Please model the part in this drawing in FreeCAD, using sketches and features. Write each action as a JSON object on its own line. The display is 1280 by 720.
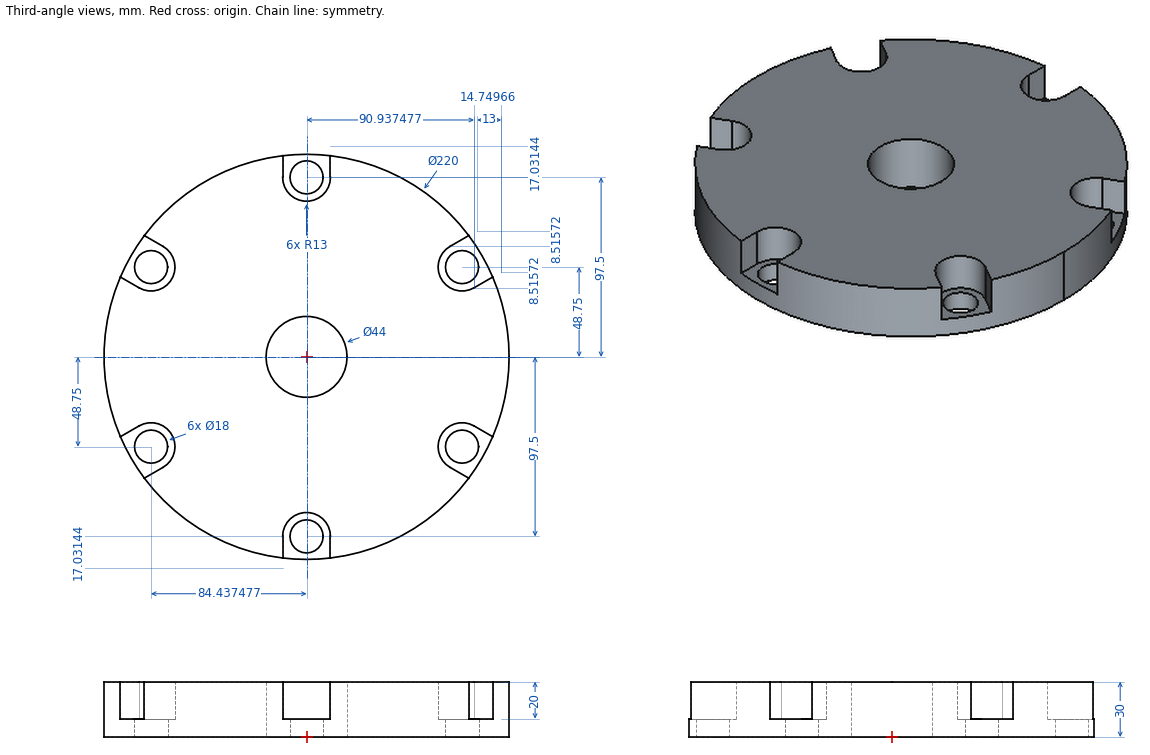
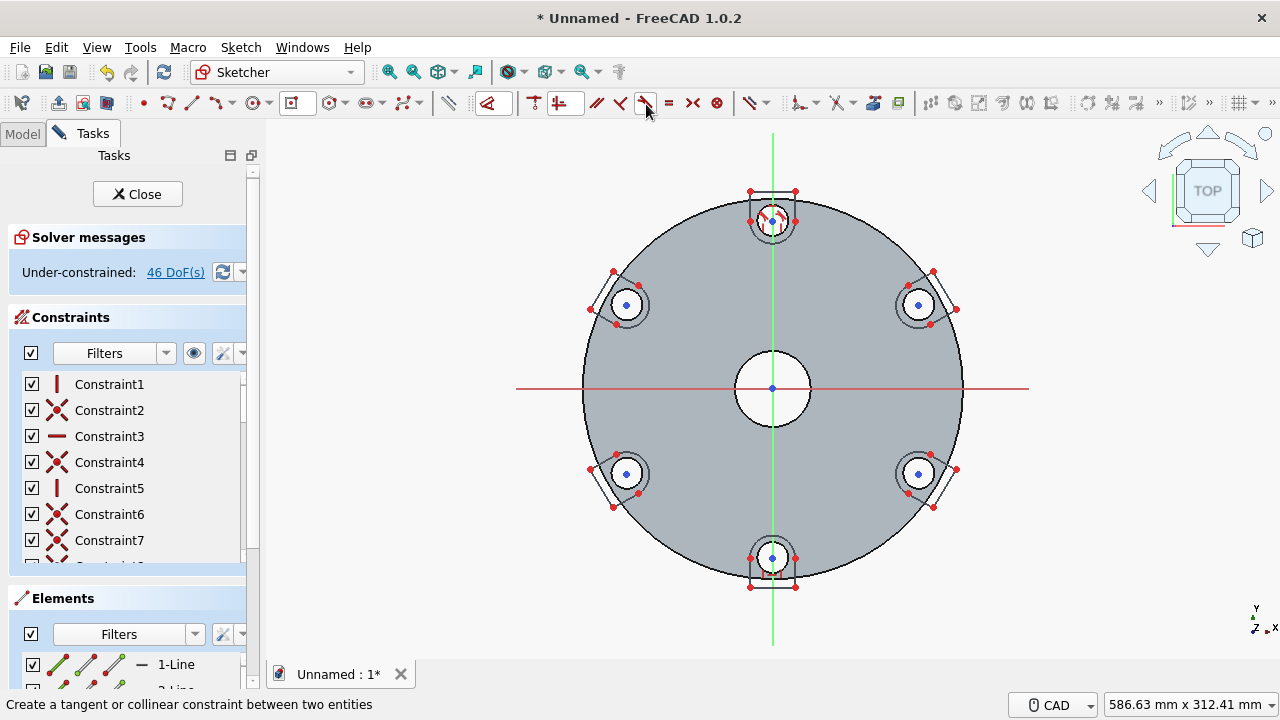
{"action": "scroll", "coordinate": [938, 320], "scroll_direction": "up", "scroll_amount": 3}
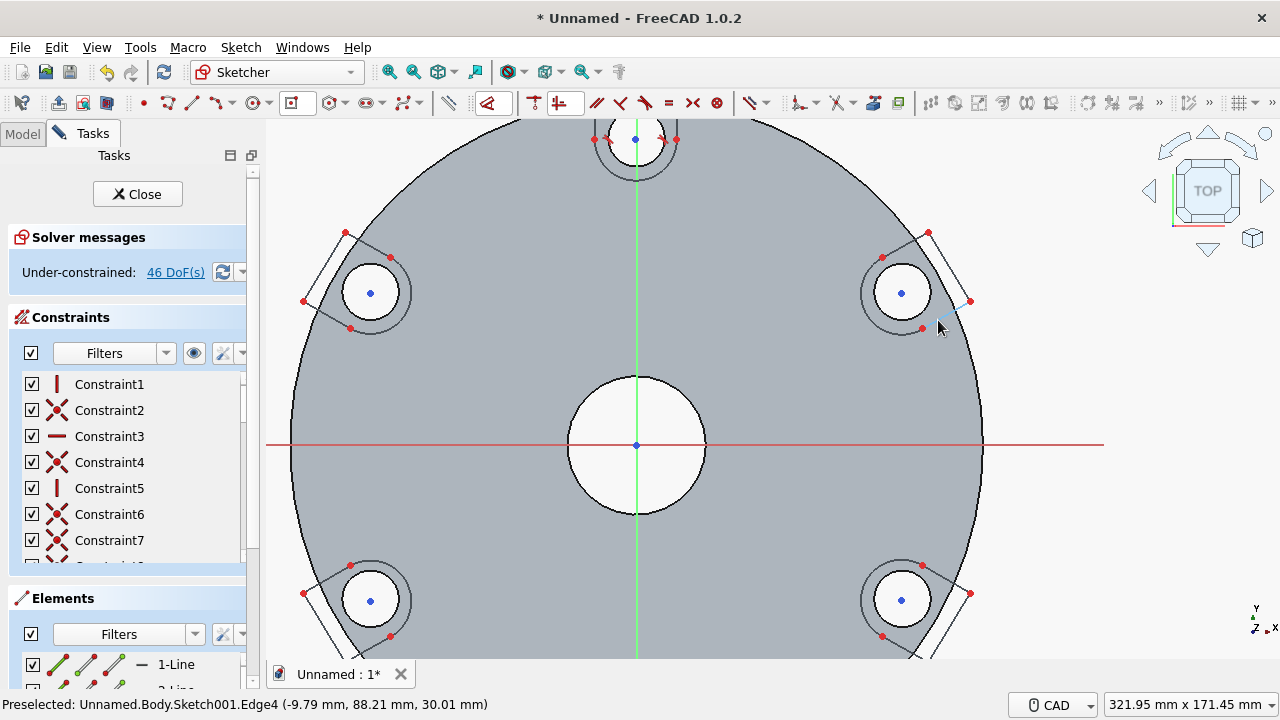
{"action": "left_click", "coordinate": [937, 321]}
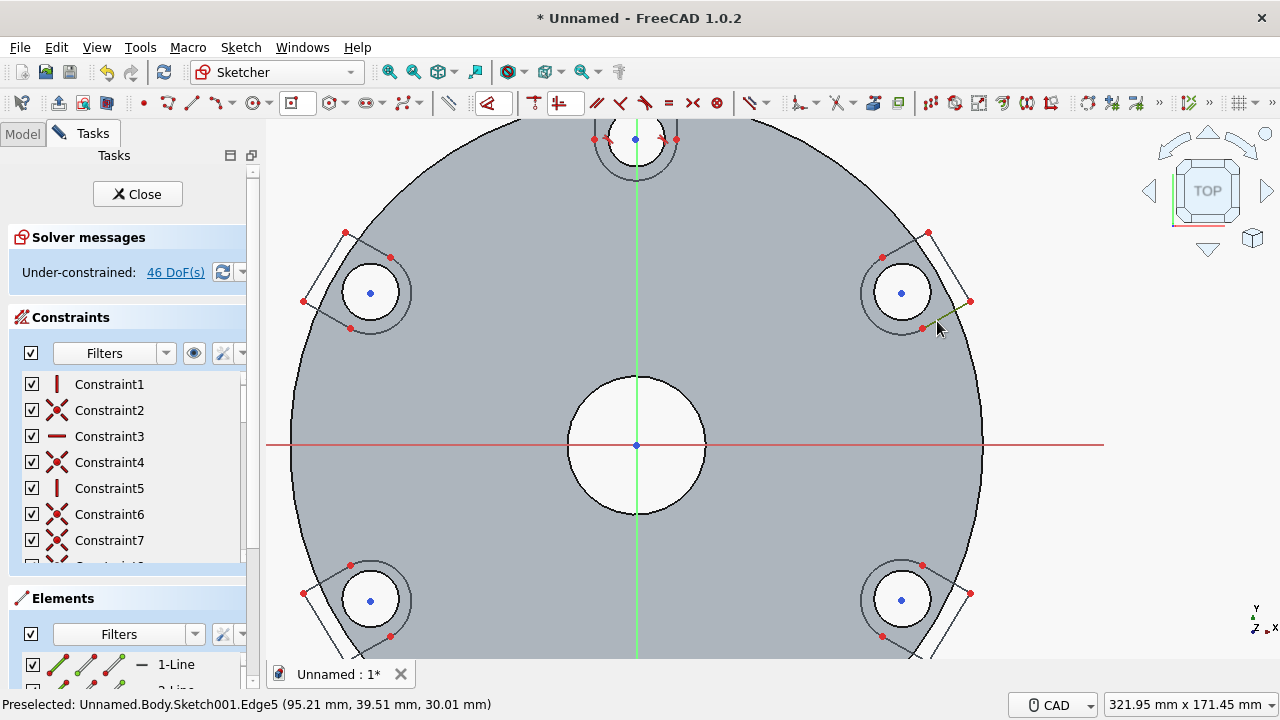
{"action": "left_click", "coordinate": [861, 289]}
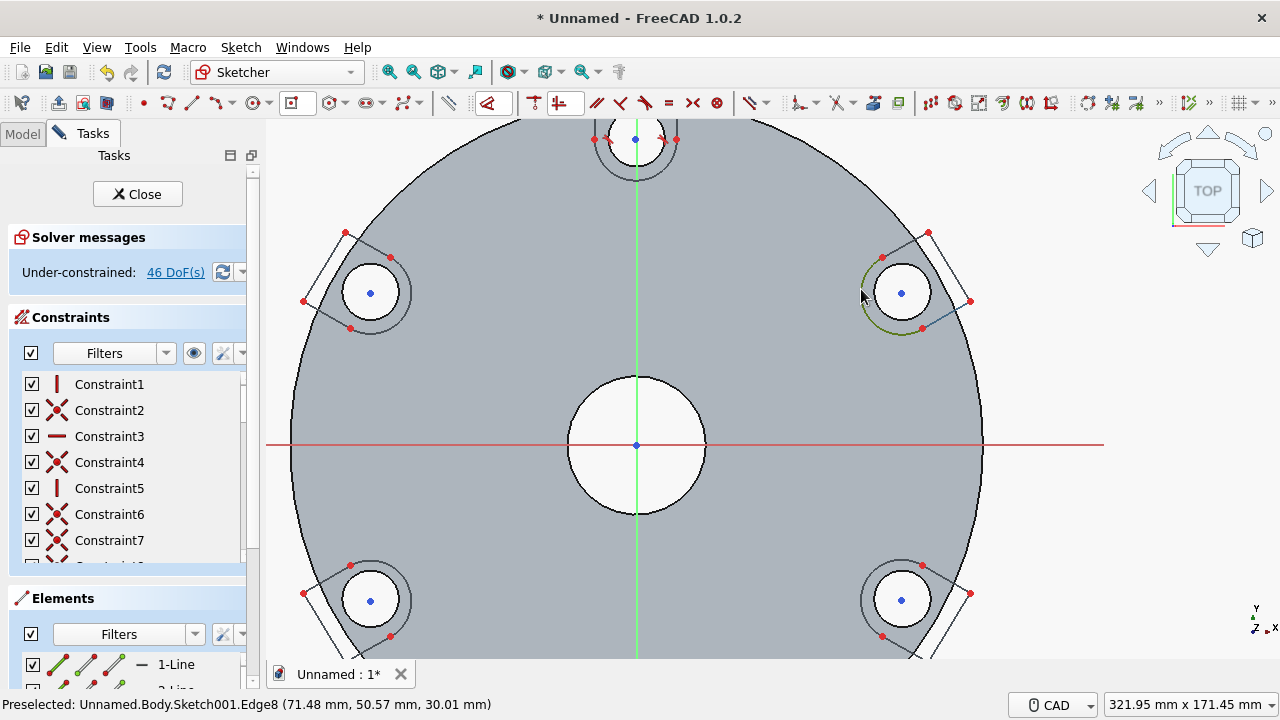
{"action": "key", "text": "t"}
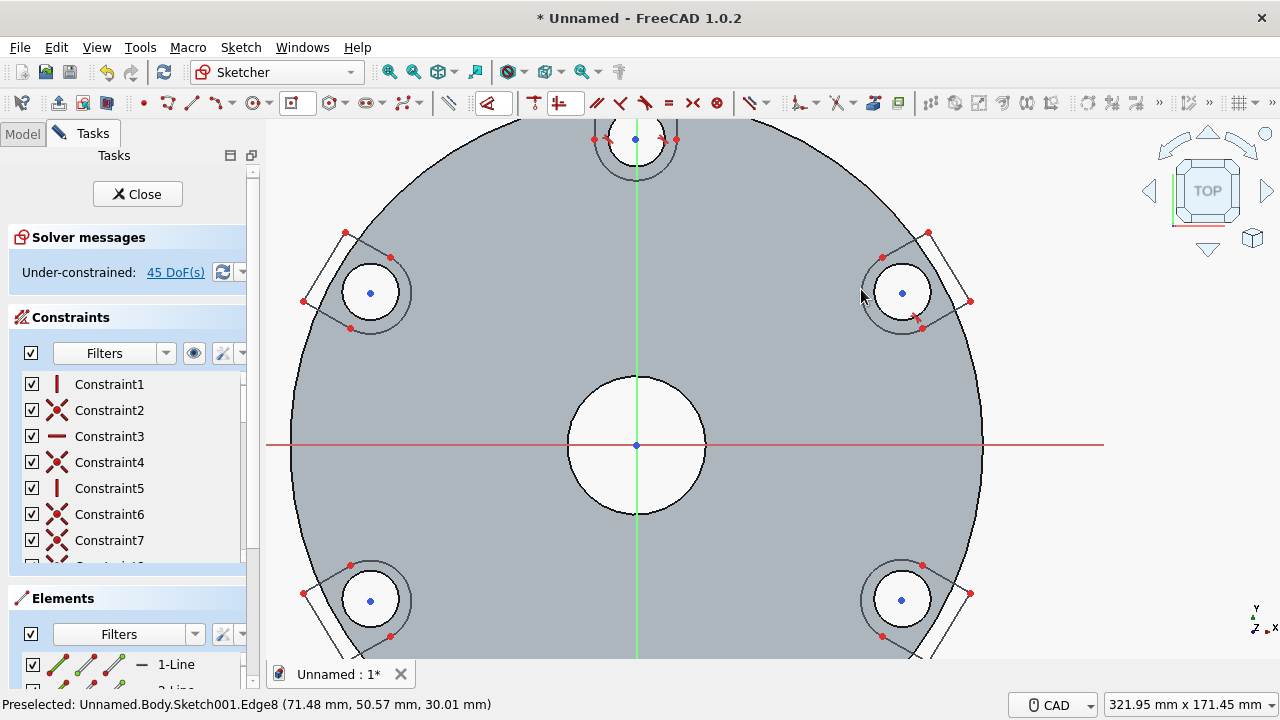
{"action": "left_click", "coordinate": [915, 240]}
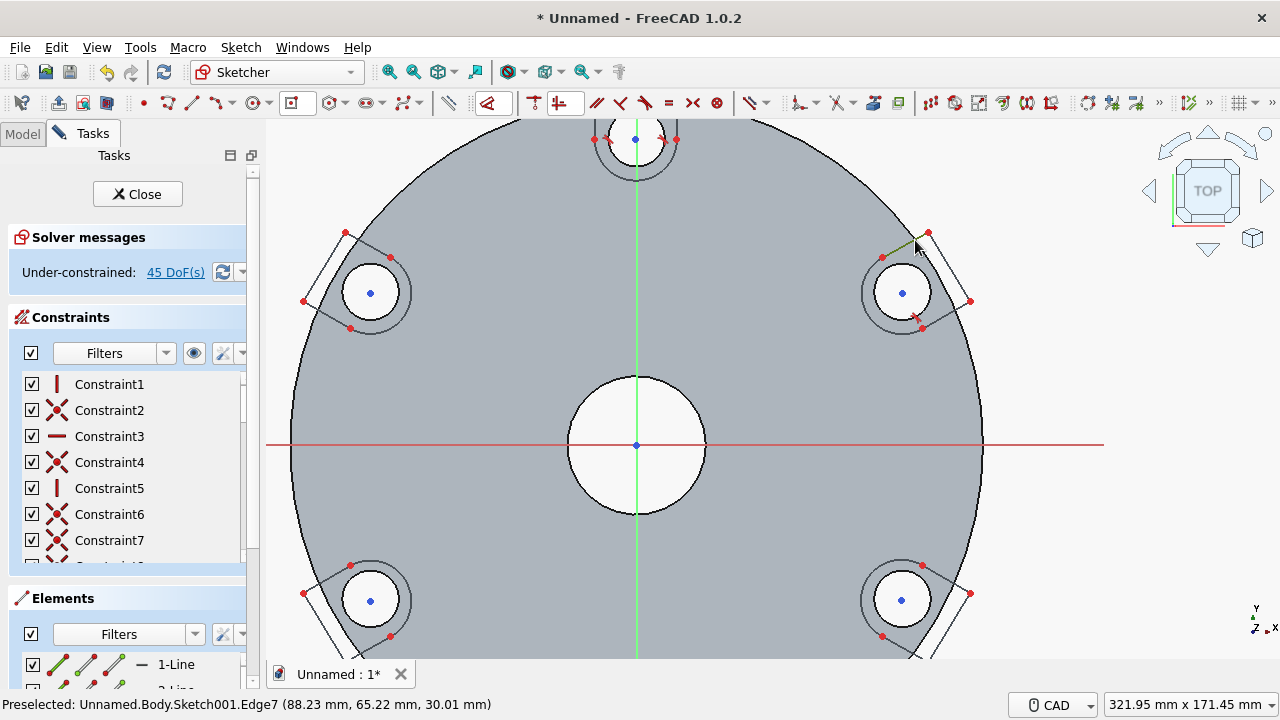
{"action": "left_click", "coordinate": [862, 289]}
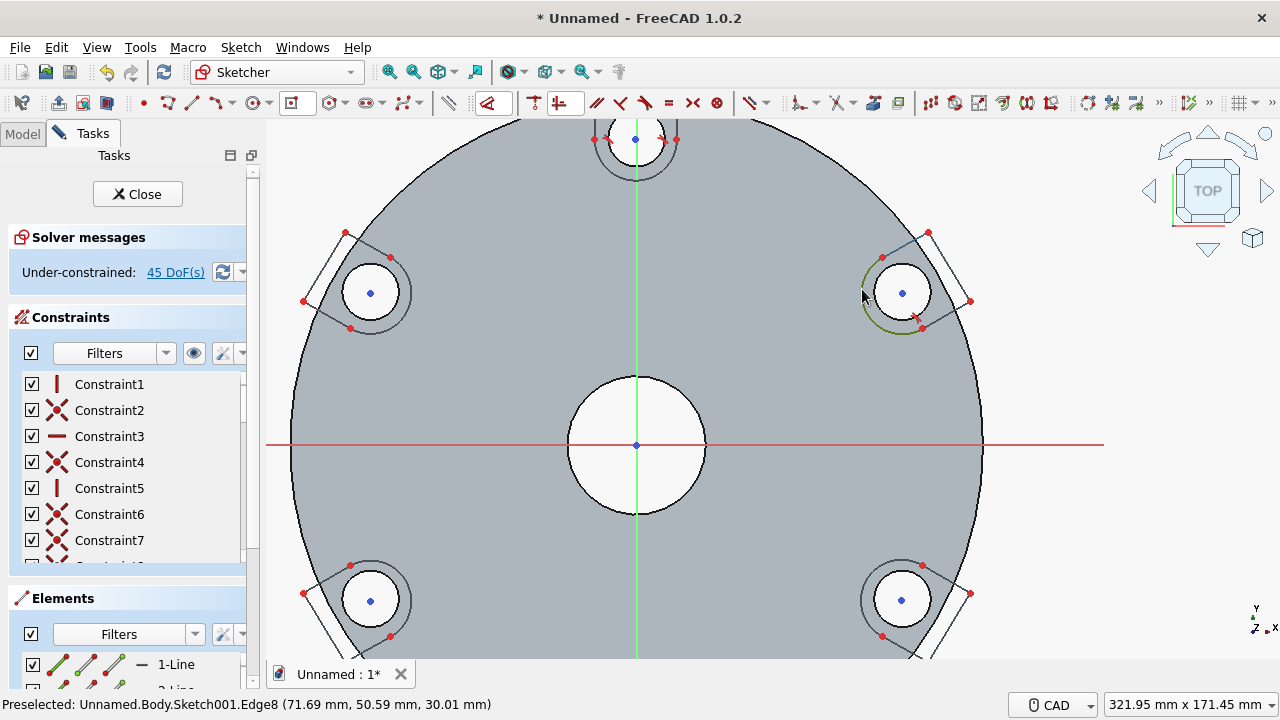
{"action": "left_click", "coordinate": [646, 104]}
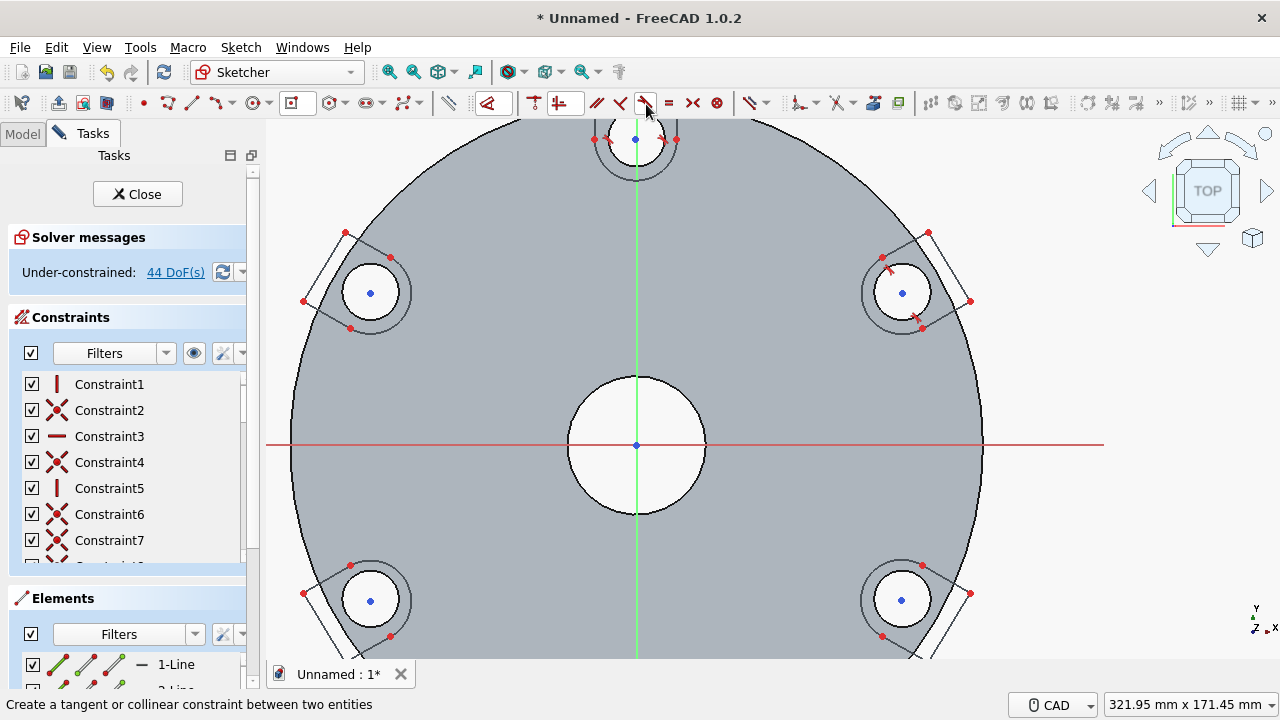
{"action": "scroll", "coordinate": [760, 343], "scroll_direction": "down", "scroll_amount": 4}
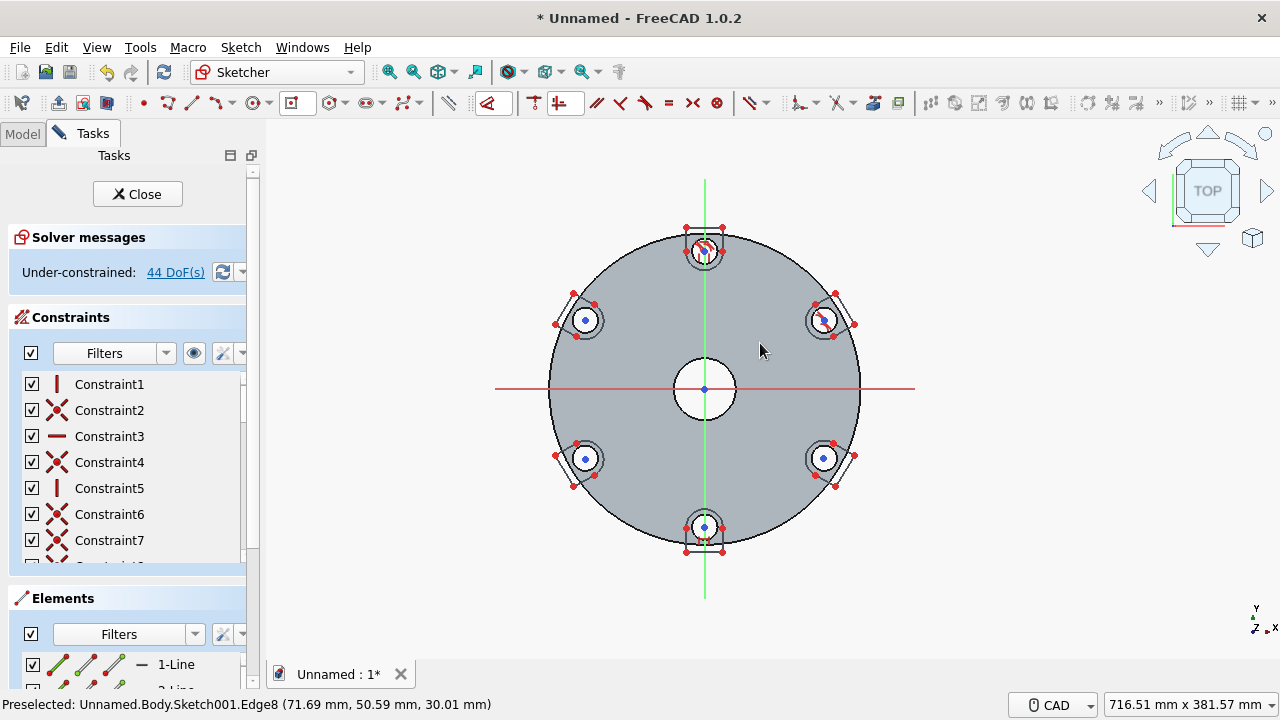
{"action": "scroll", "coordinate": [822, 479], "scroll_direction": "up", "scroll_amount": 4}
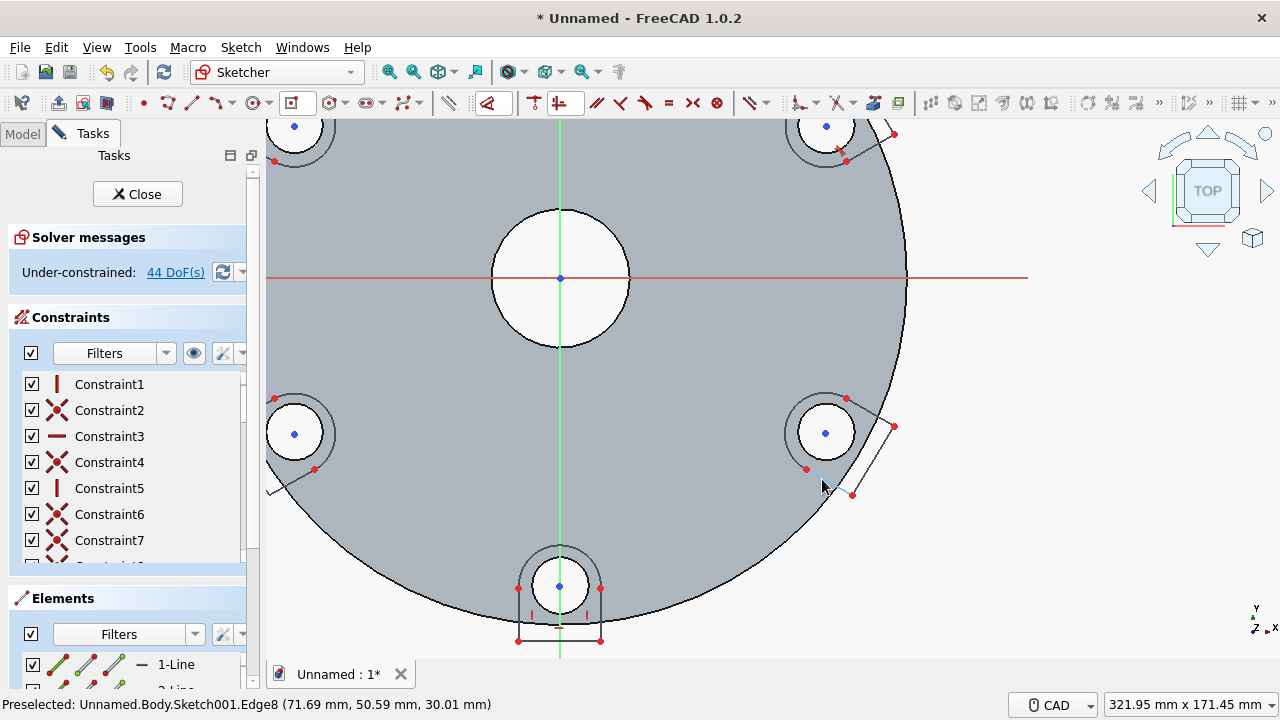
{"action": "left_click", "coordinate": [820, 477]}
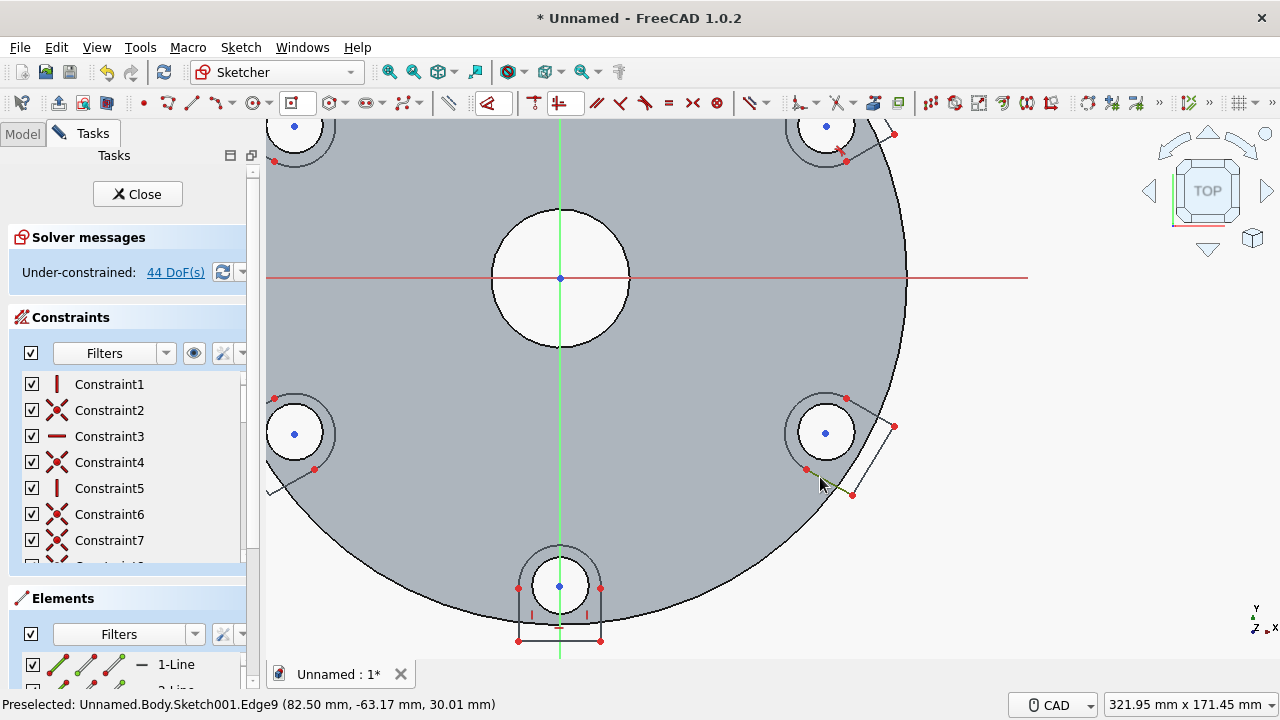
{"action": "left_click", "coordinate": [809, 396]}